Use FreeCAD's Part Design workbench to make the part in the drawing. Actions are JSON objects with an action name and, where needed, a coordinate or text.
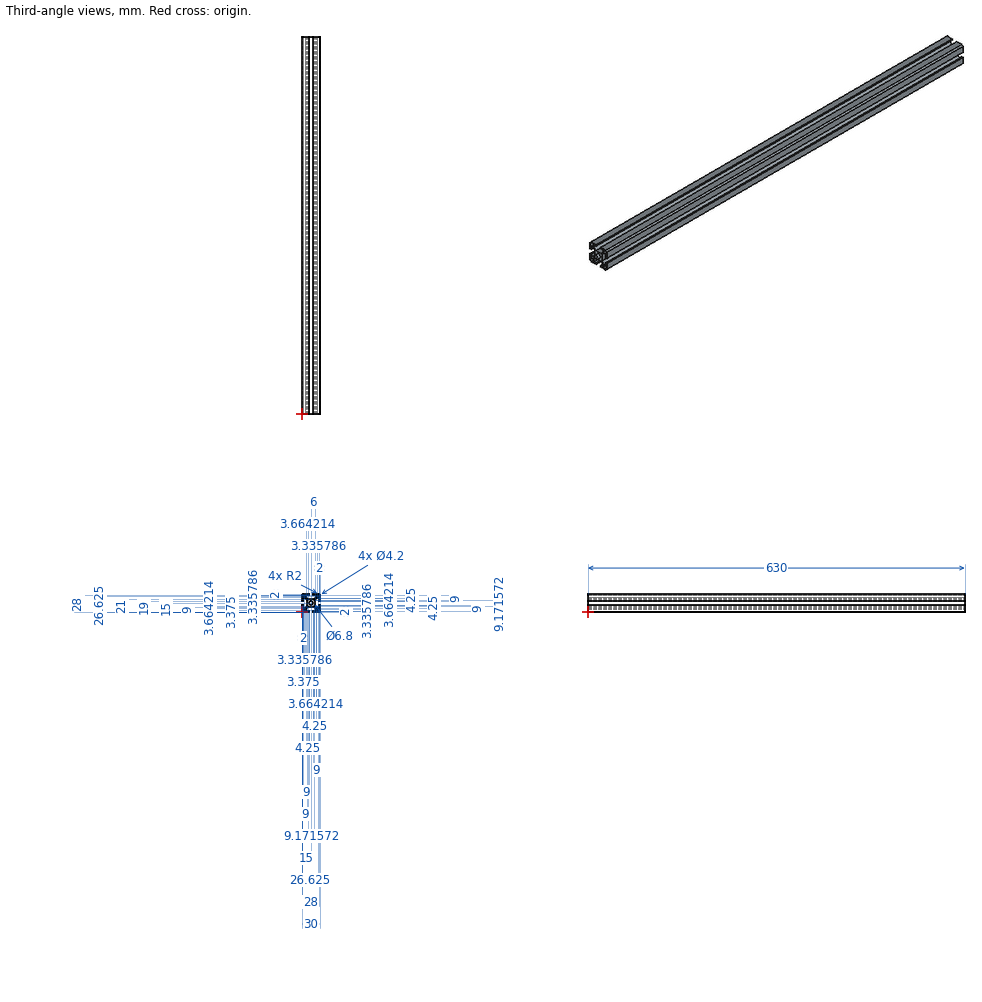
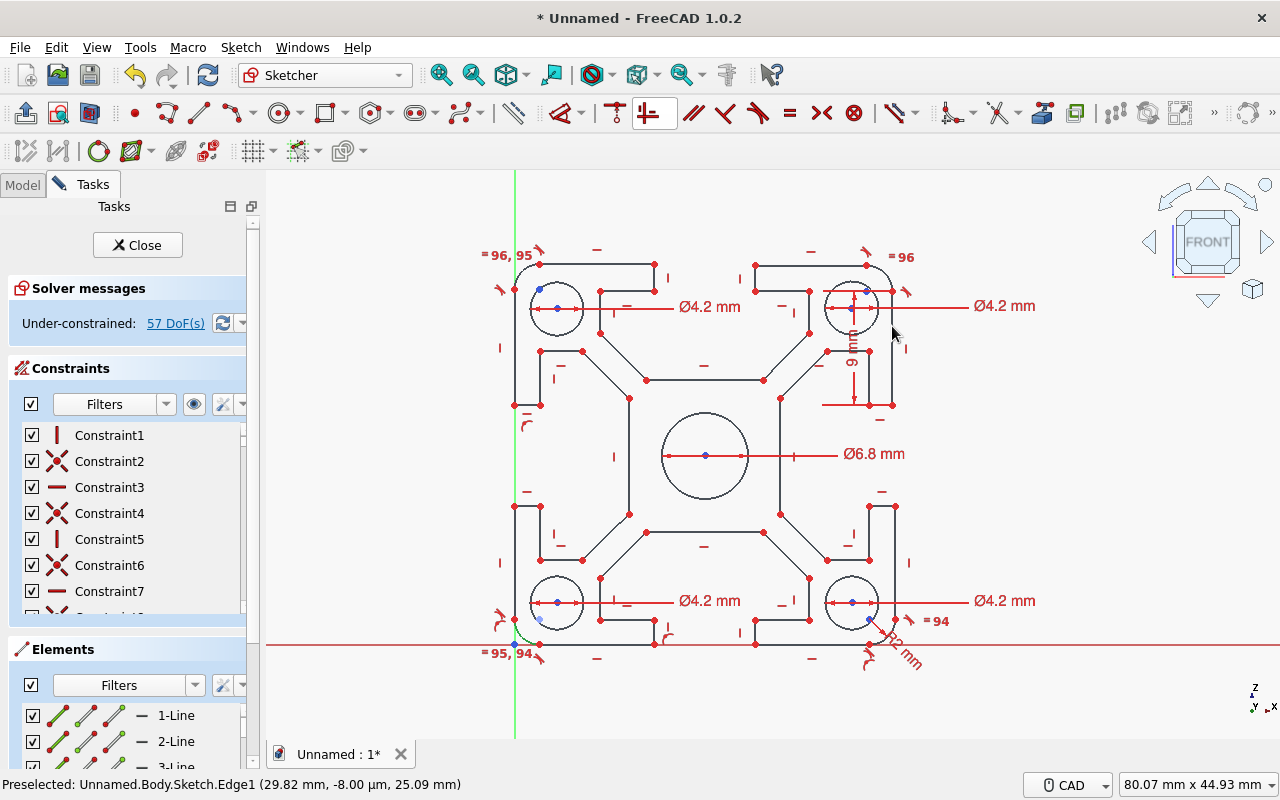
{"action": "scroll", "coordinate": [883, 405], "scroll_direction": "up", "scroll_amount": 3}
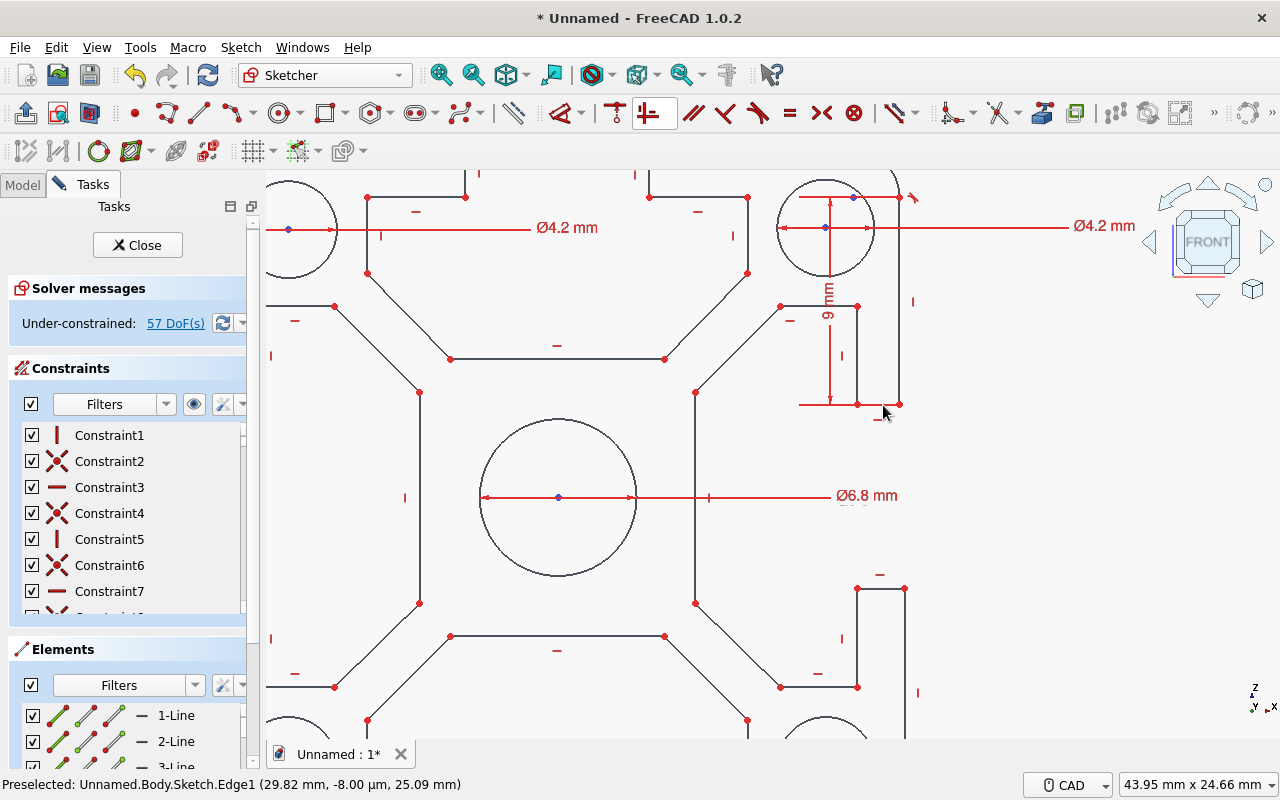
{"action": "left_click", "coordinate": [883, 405]}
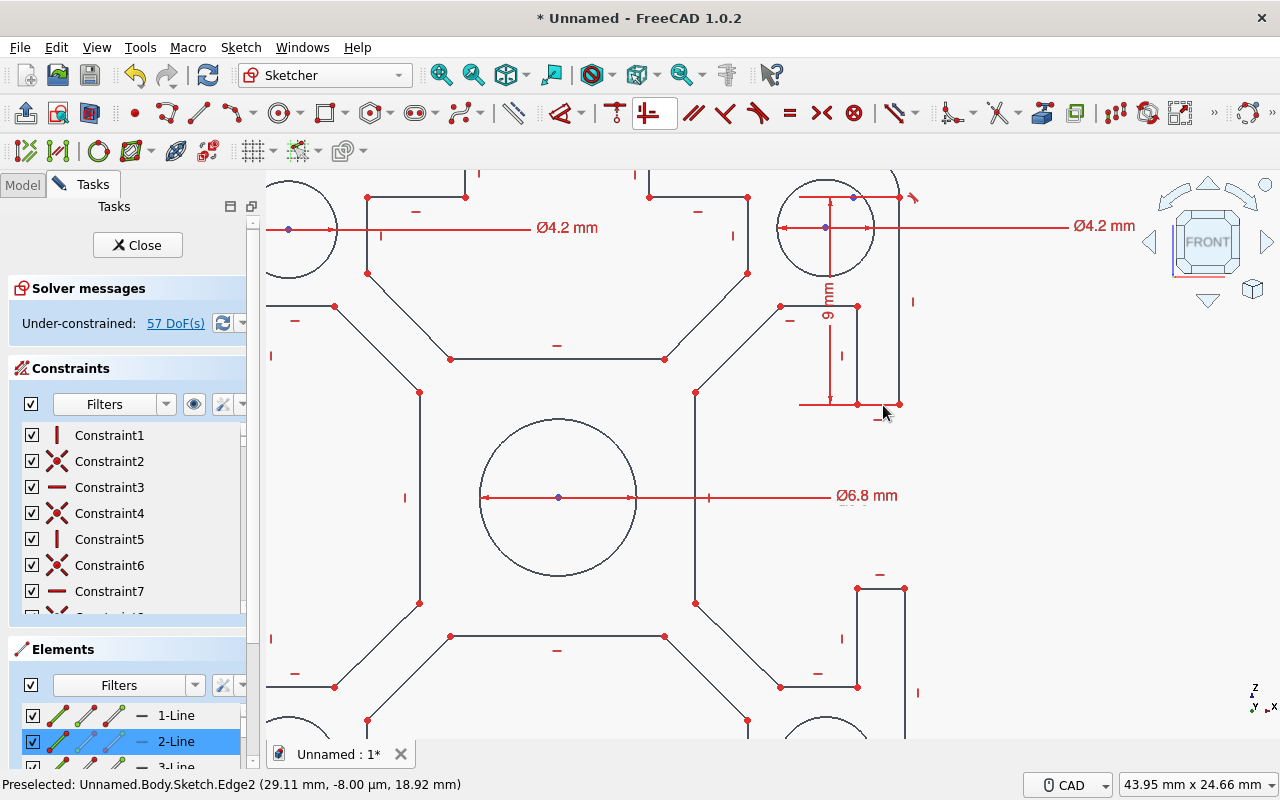
{"action": "left_click", "coordinate": [584, 114]}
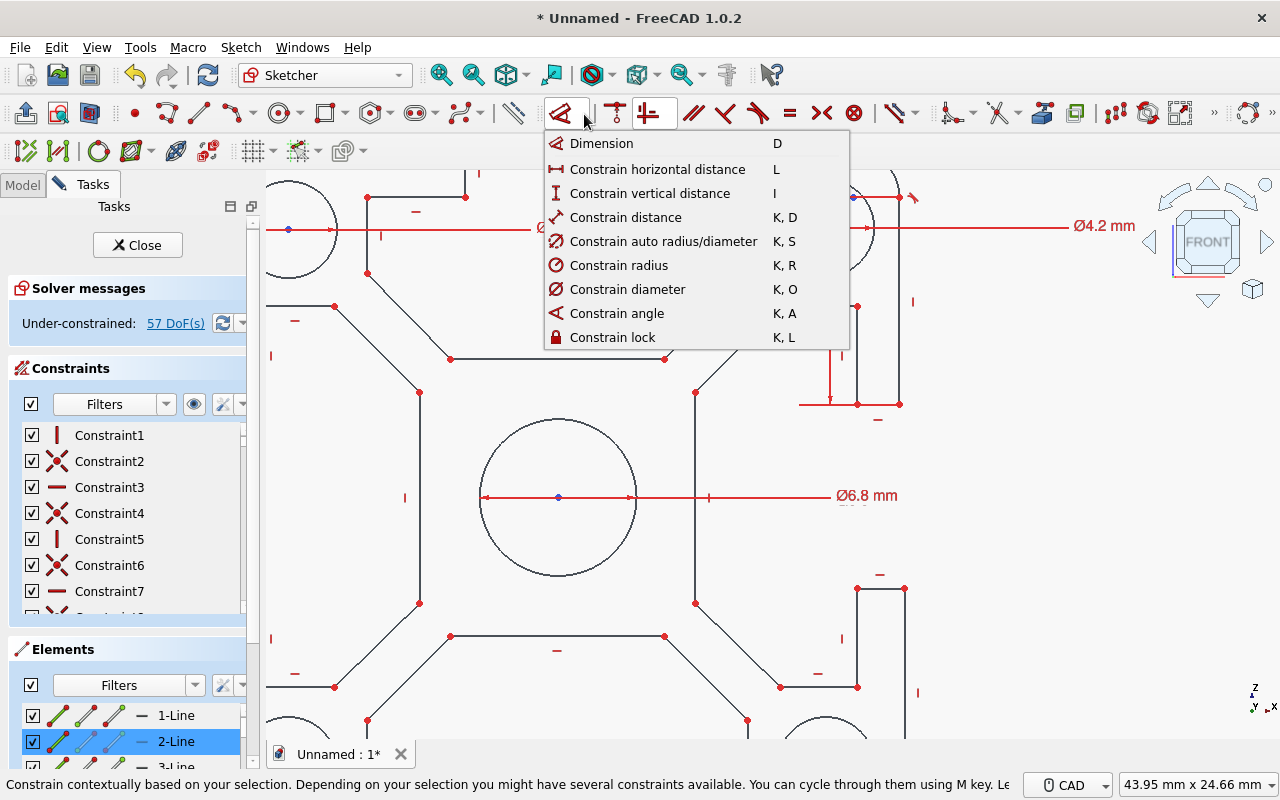
{"action": "left_click", "coordinate": [697, 169]}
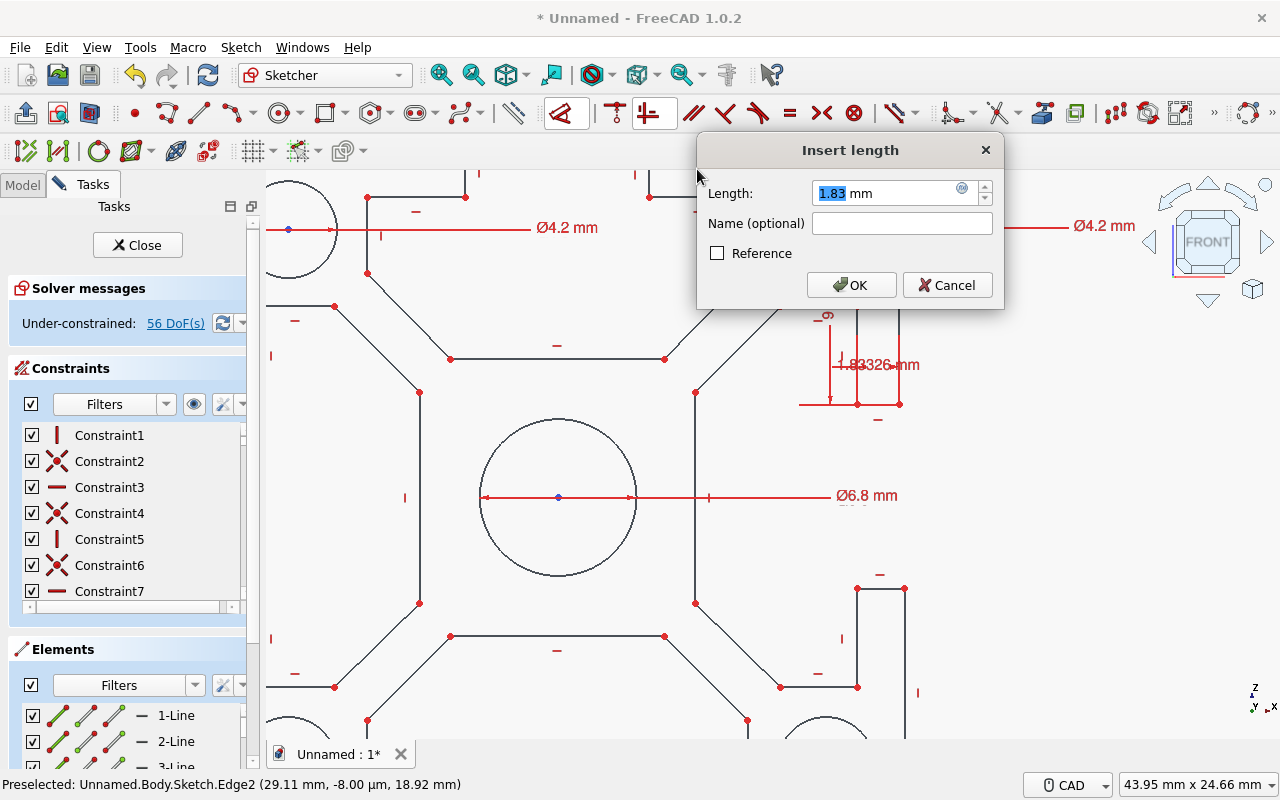
{"action": "type", "text": "2"}
{"action": "key", "text": "Return"}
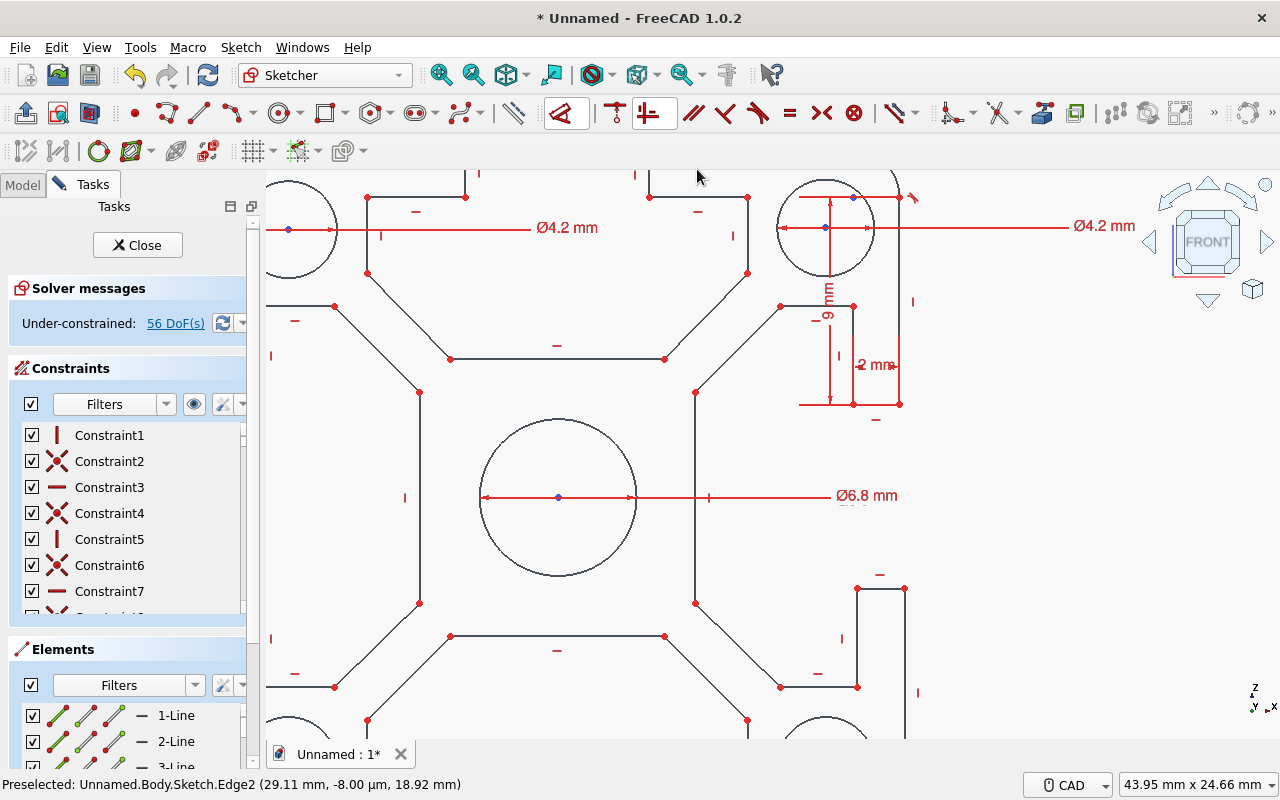
{"action": "left_click", "coordinate": [871, 589]}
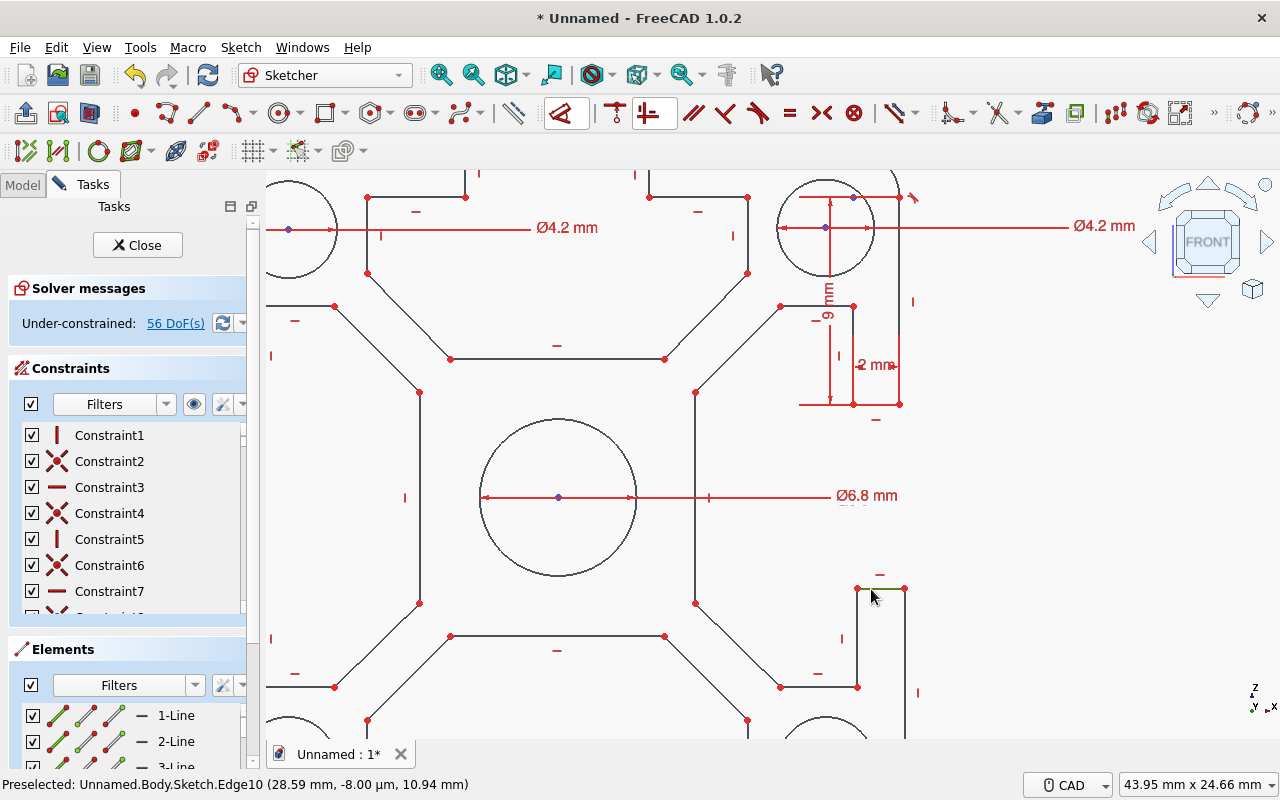
{"action": "key", "text": "l"}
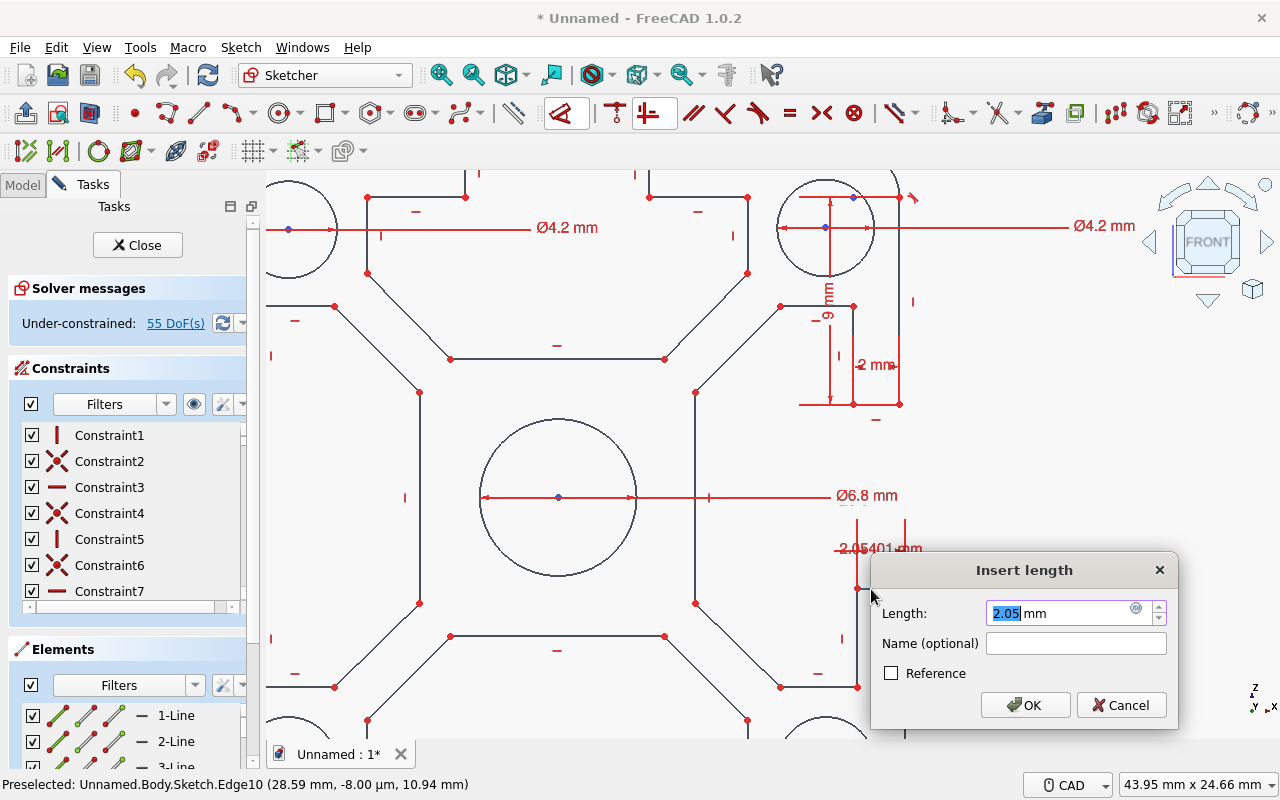
{"action": "type", "text": "2"}
{"action": "key", "text": "Return"}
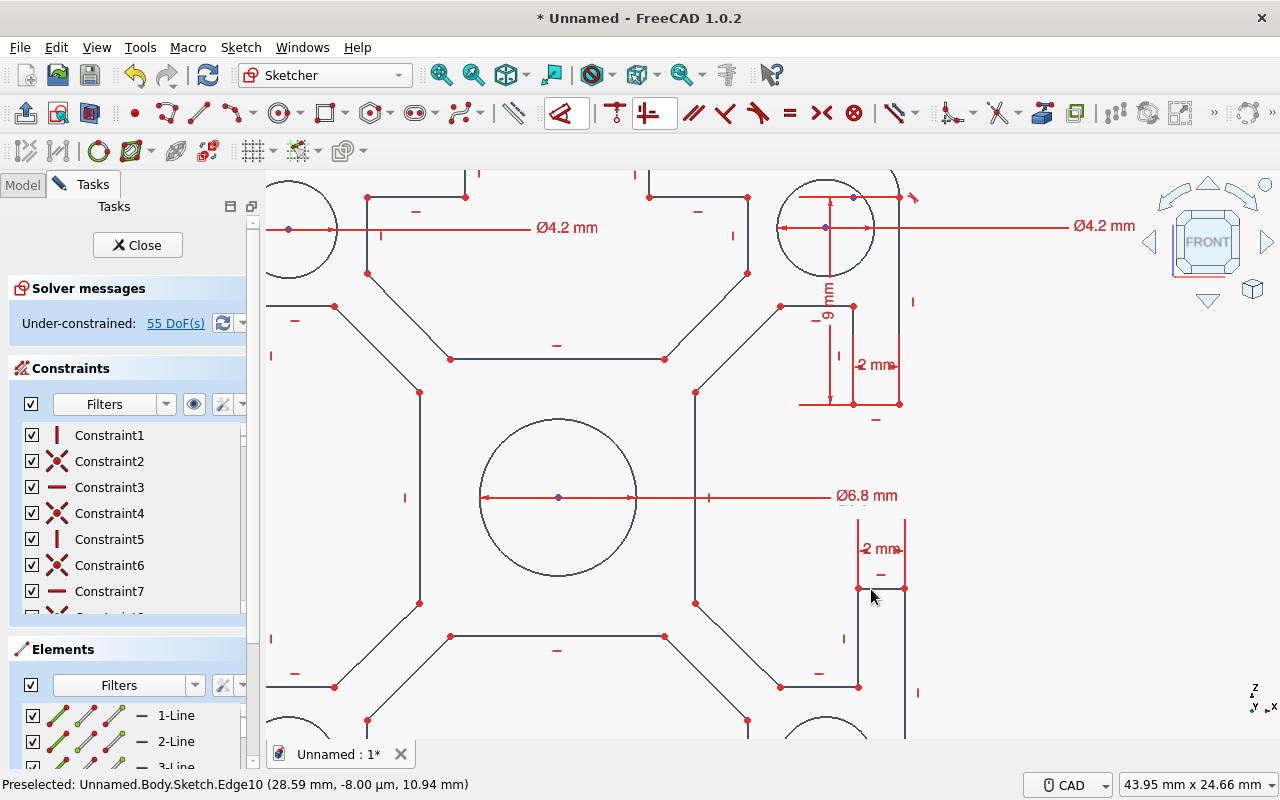
{"action": "left_click", "coordinate": [905, 651]}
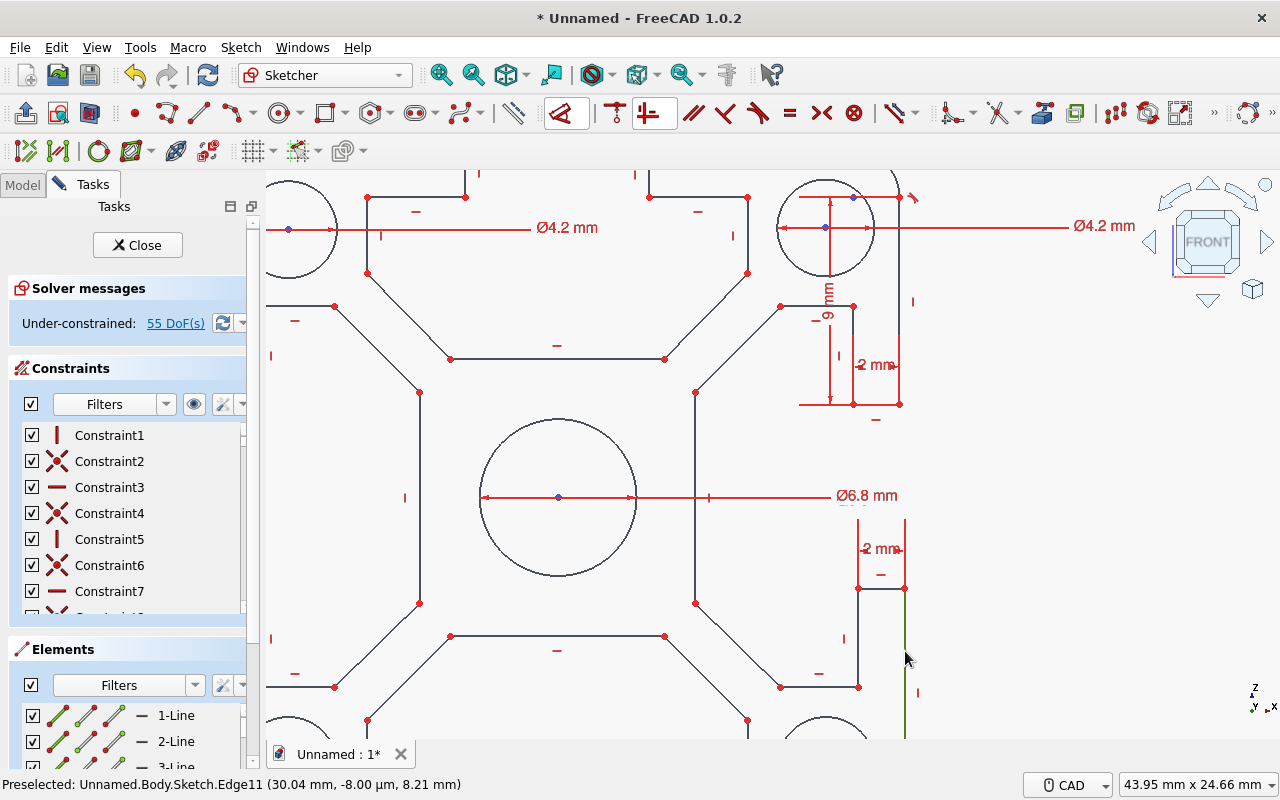
{"action": "key", "text": "i"}